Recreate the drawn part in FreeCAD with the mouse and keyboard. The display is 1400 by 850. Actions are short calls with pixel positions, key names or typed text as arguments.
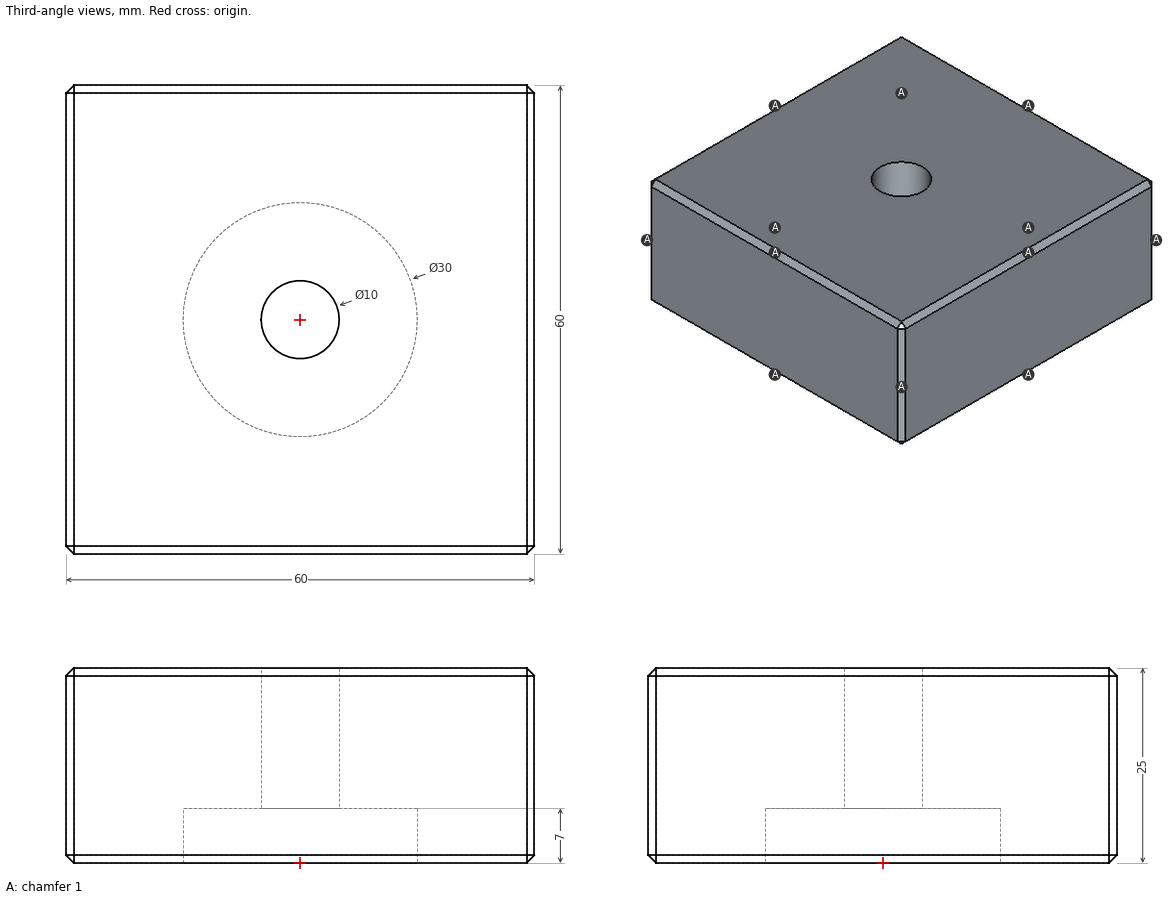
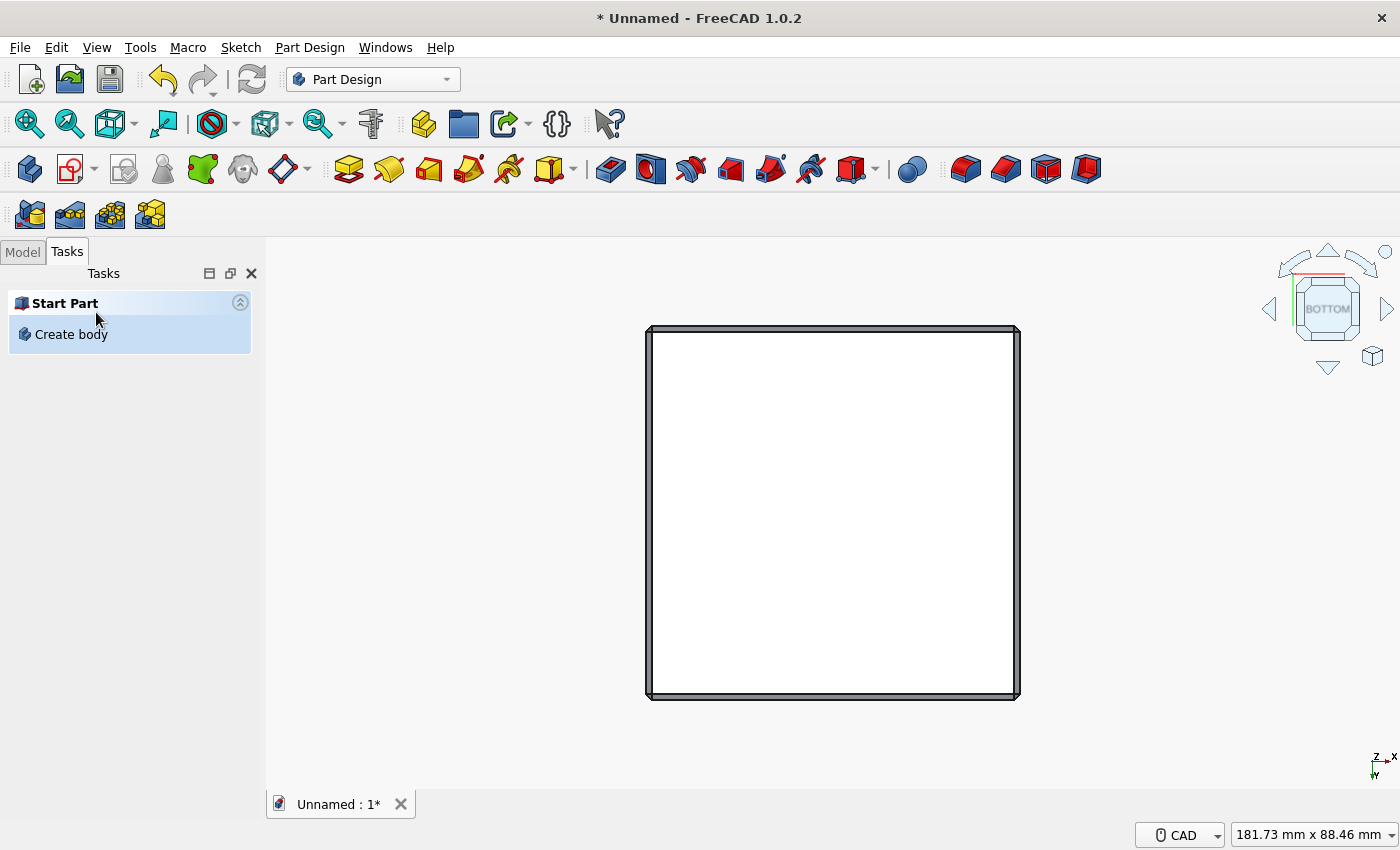
click(833, 512)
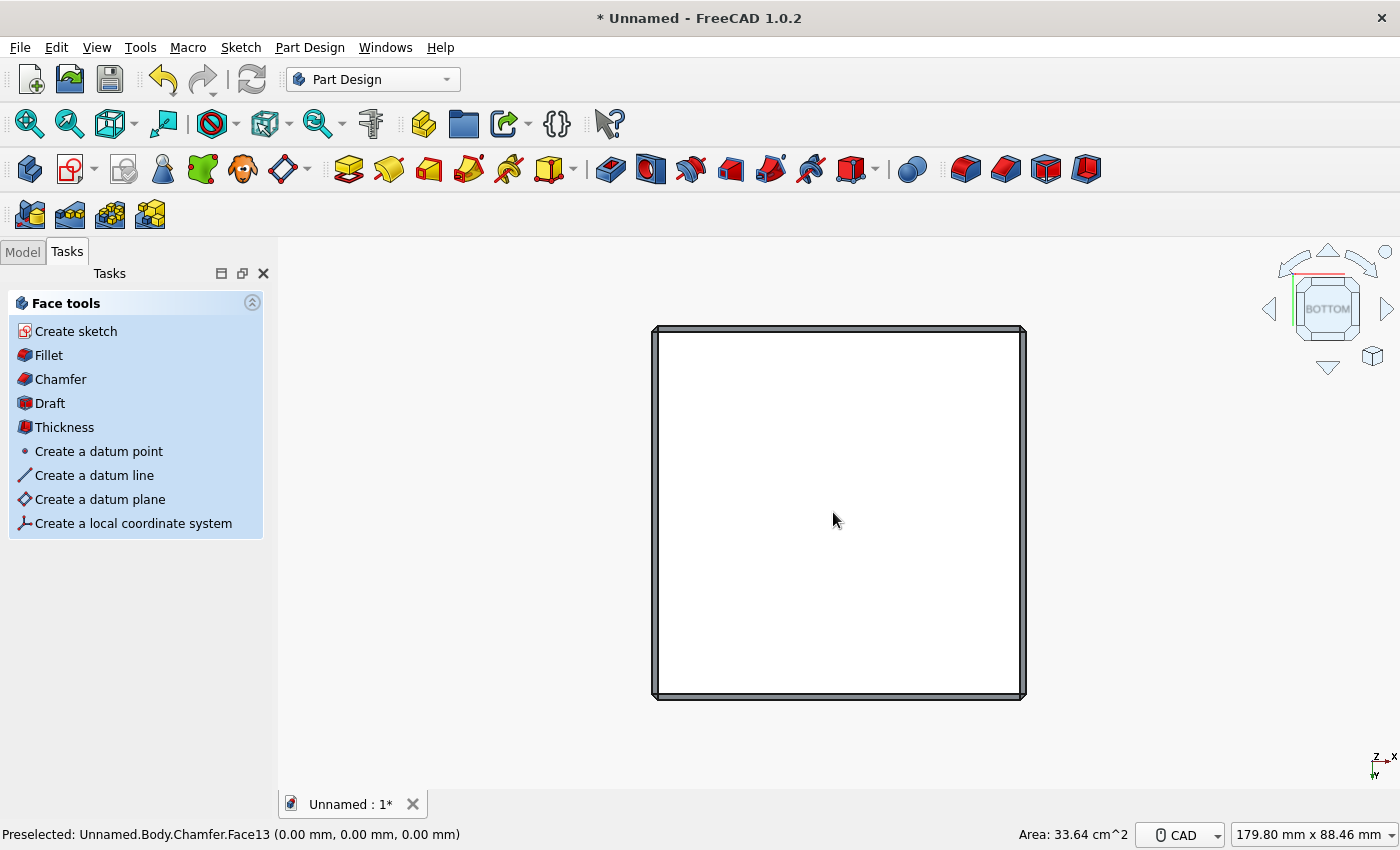
click(70, 170)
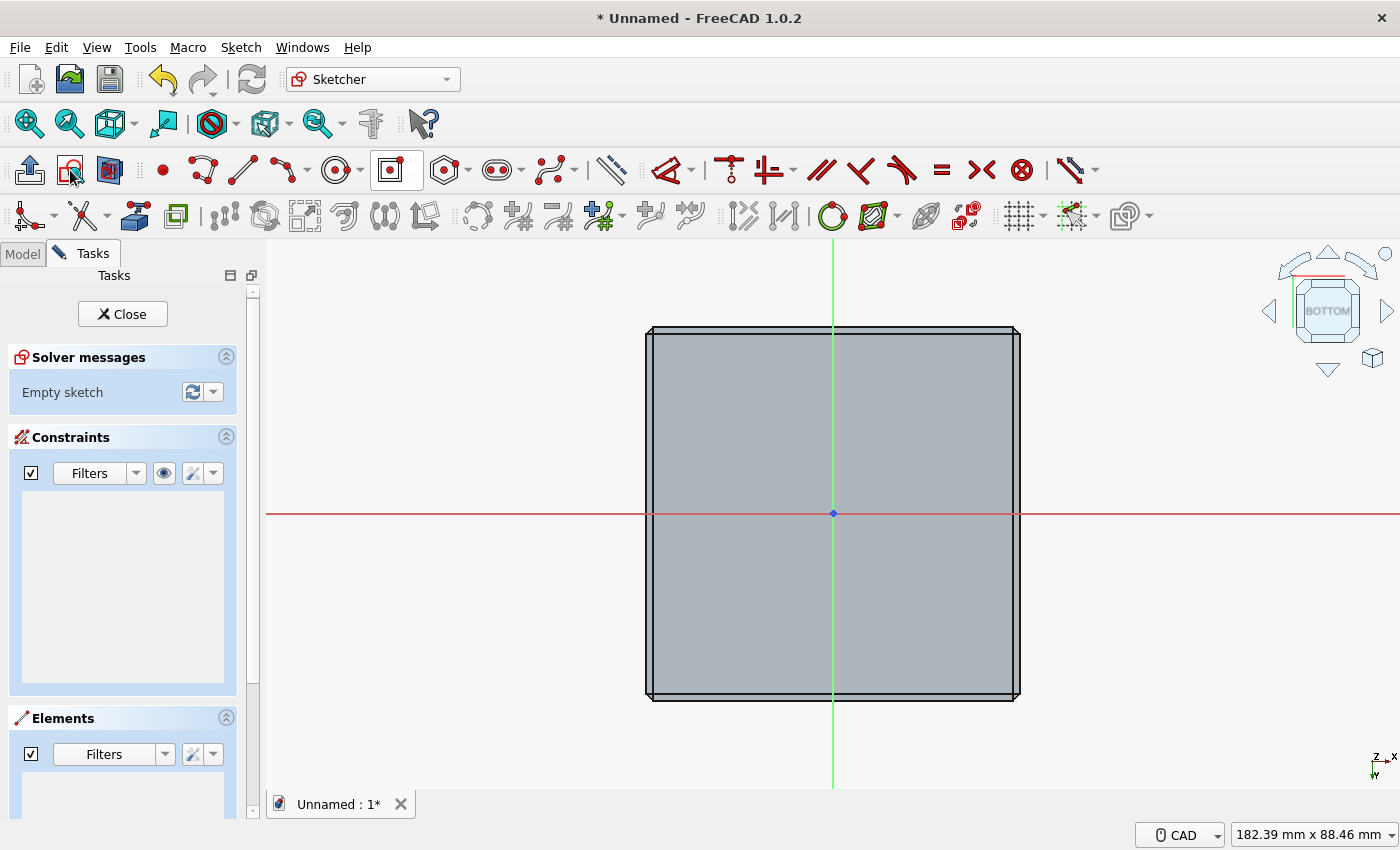
scroll(916, 514, up, 3)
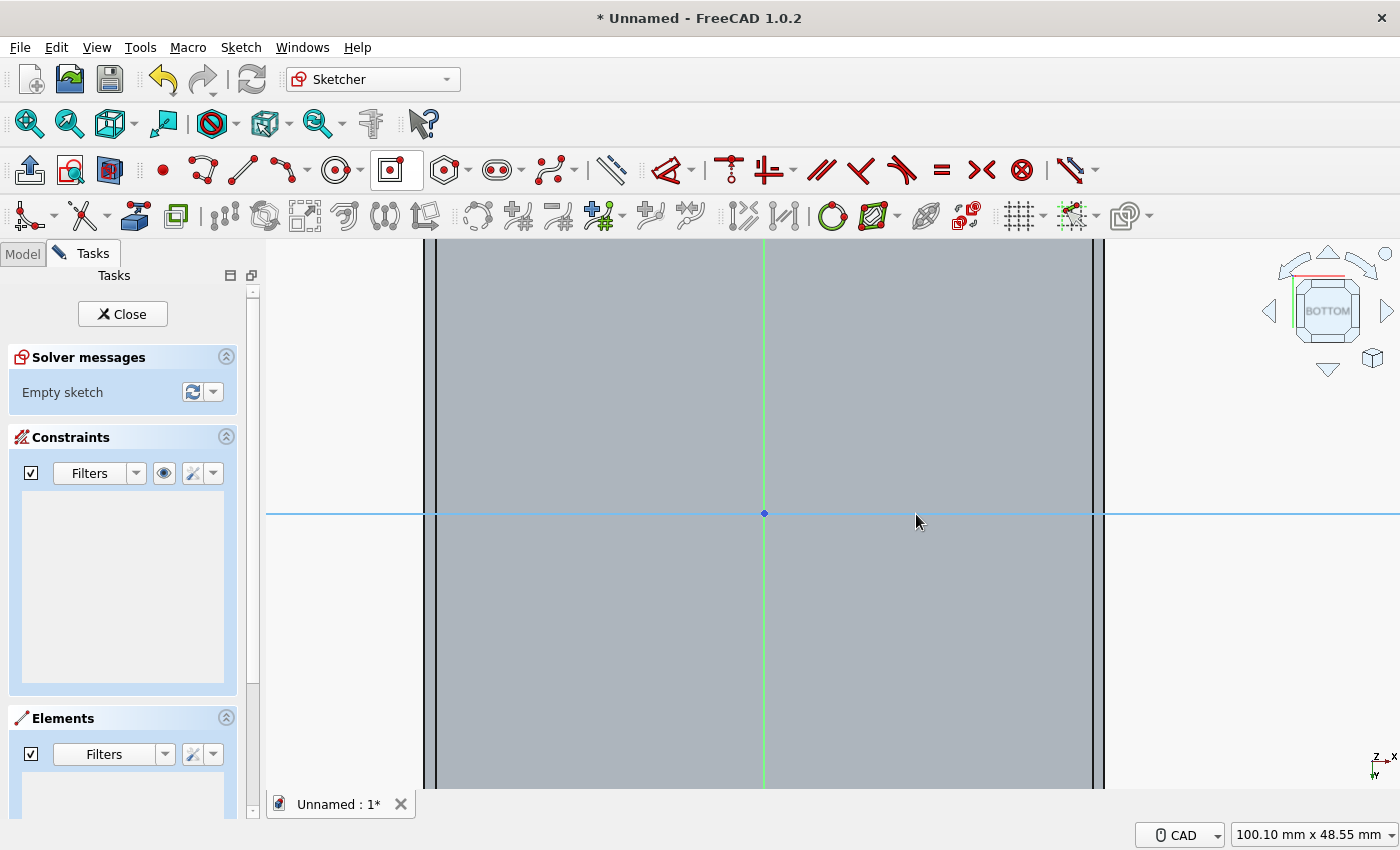
click(336, 170)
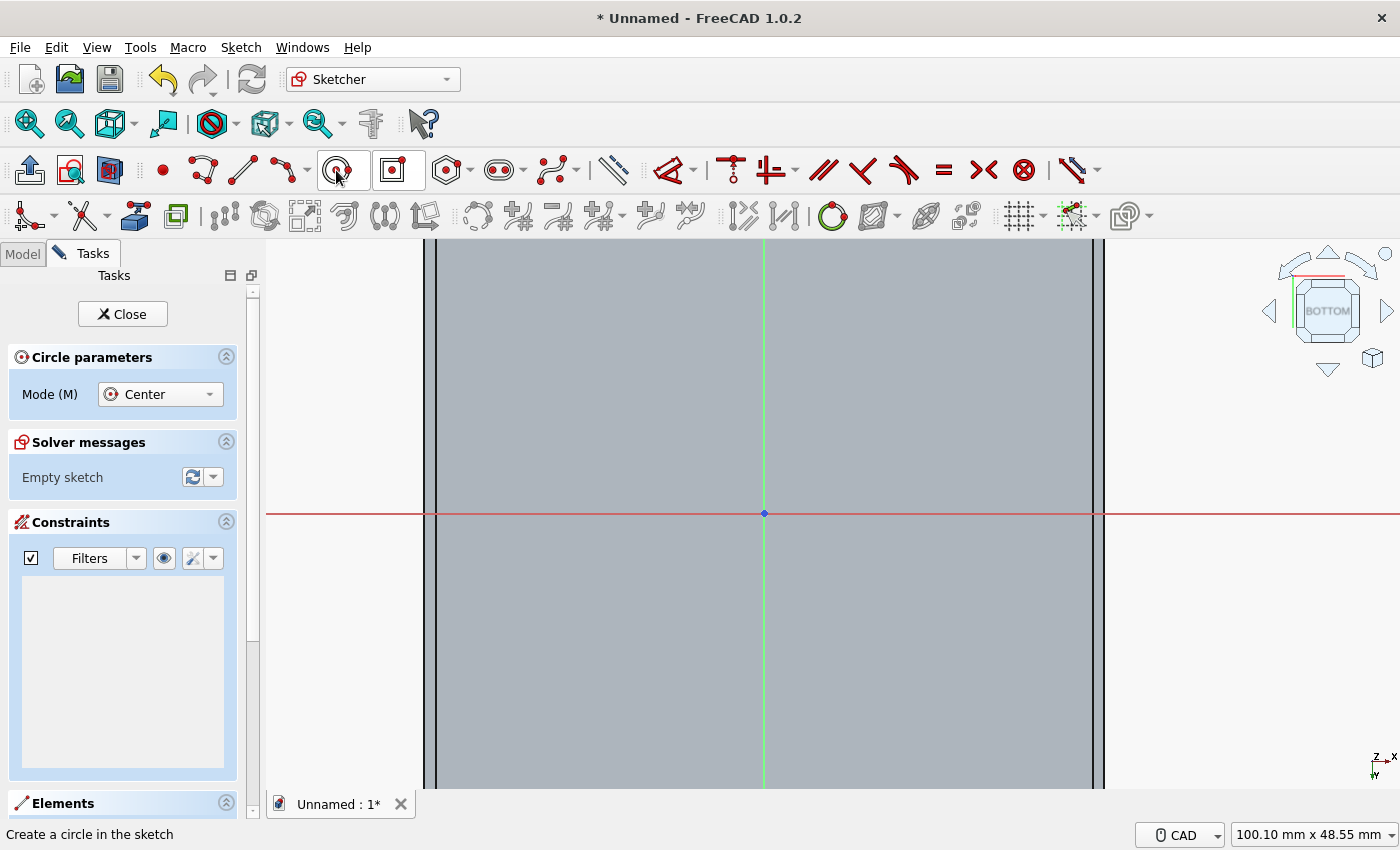
click(764, 514)
move(884, 393)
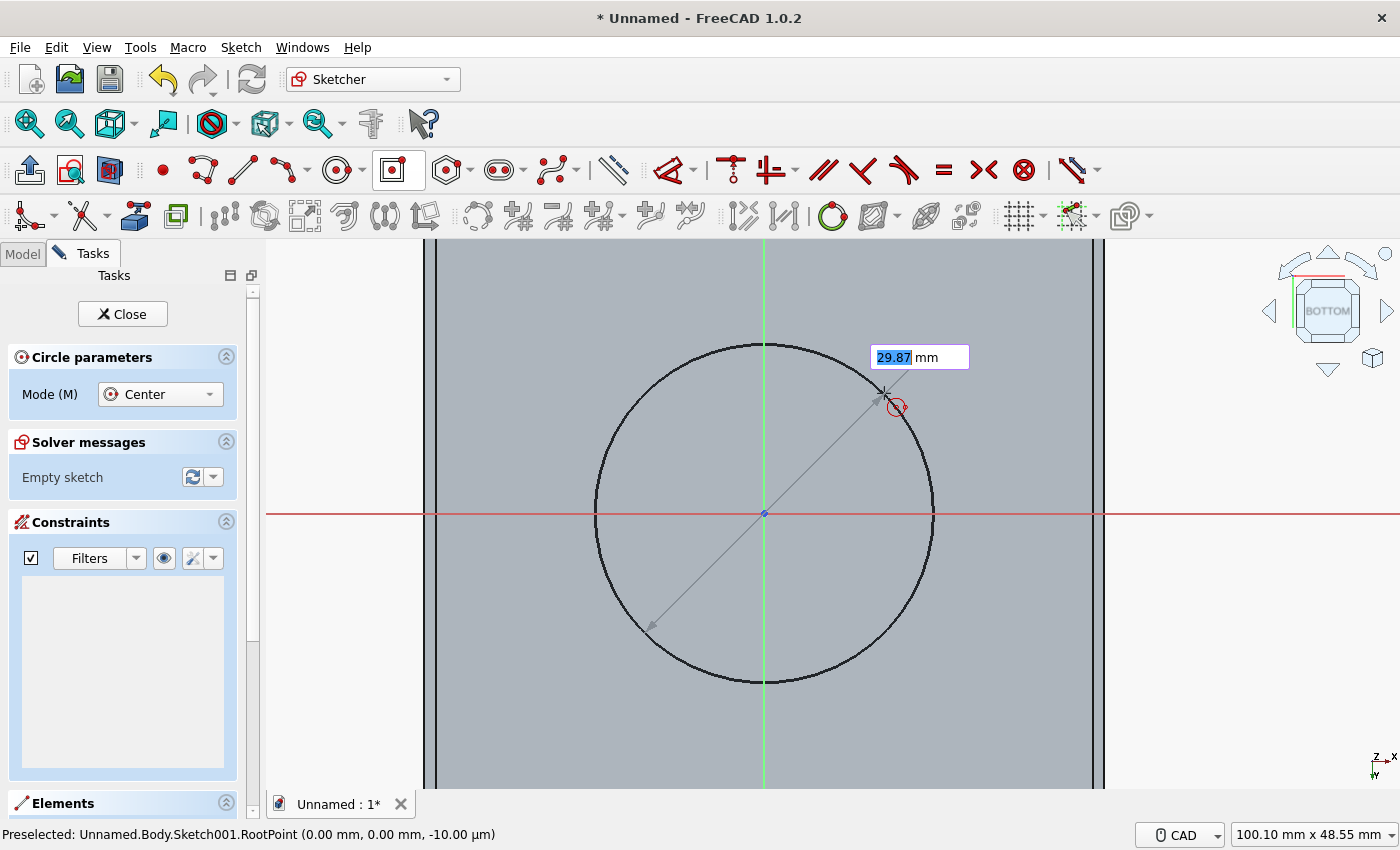
text(30)
key(Return)
key(Escape)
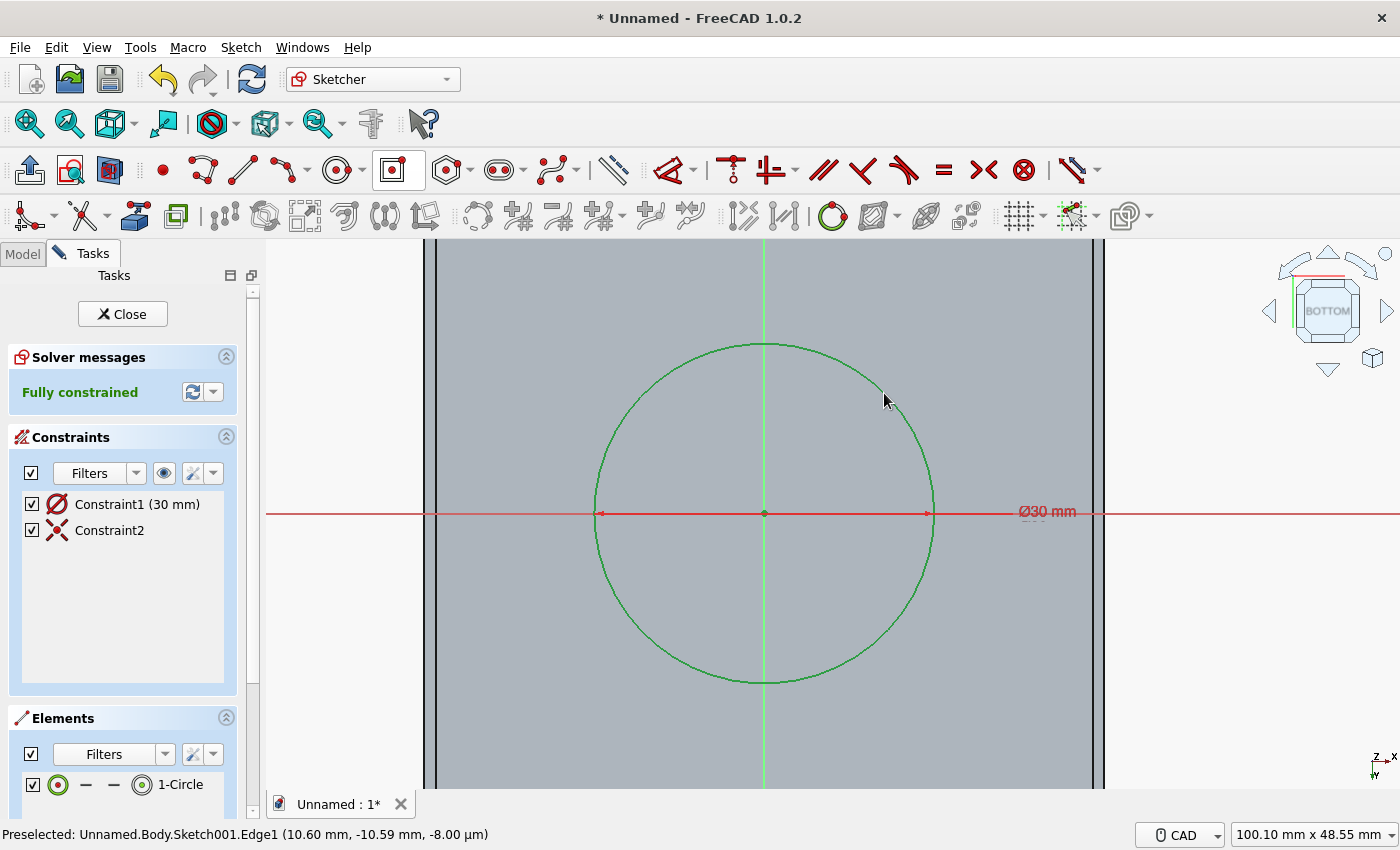
click(123, 314)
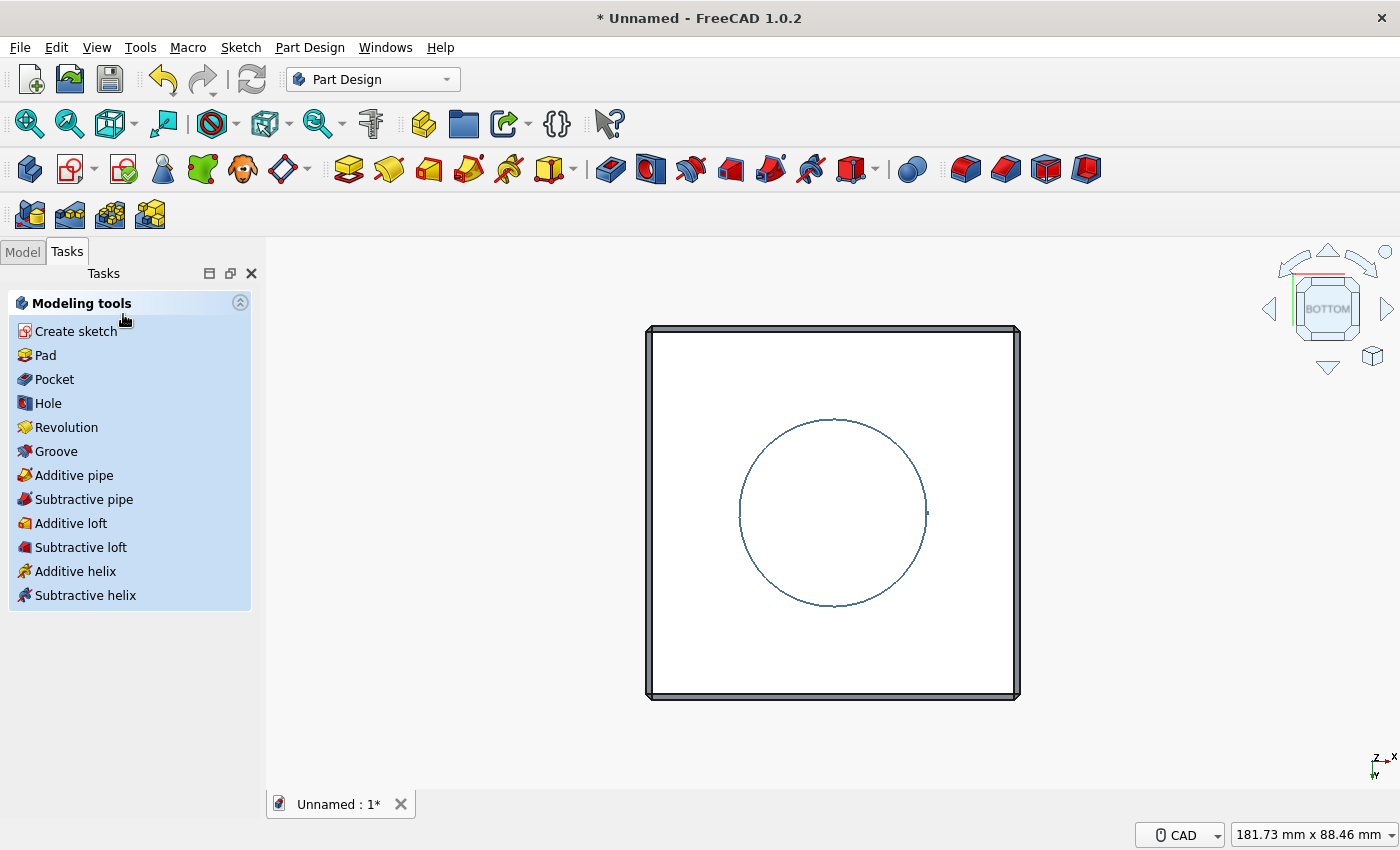
click(612, 170)